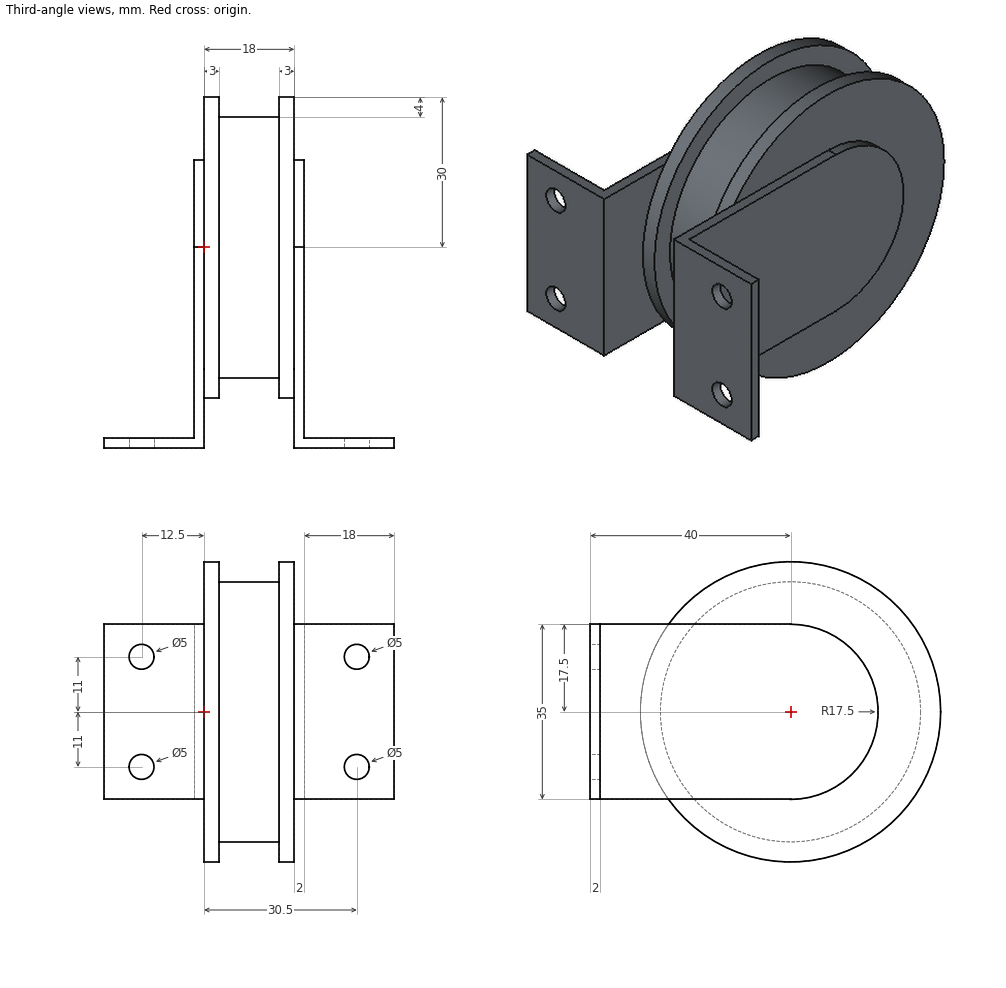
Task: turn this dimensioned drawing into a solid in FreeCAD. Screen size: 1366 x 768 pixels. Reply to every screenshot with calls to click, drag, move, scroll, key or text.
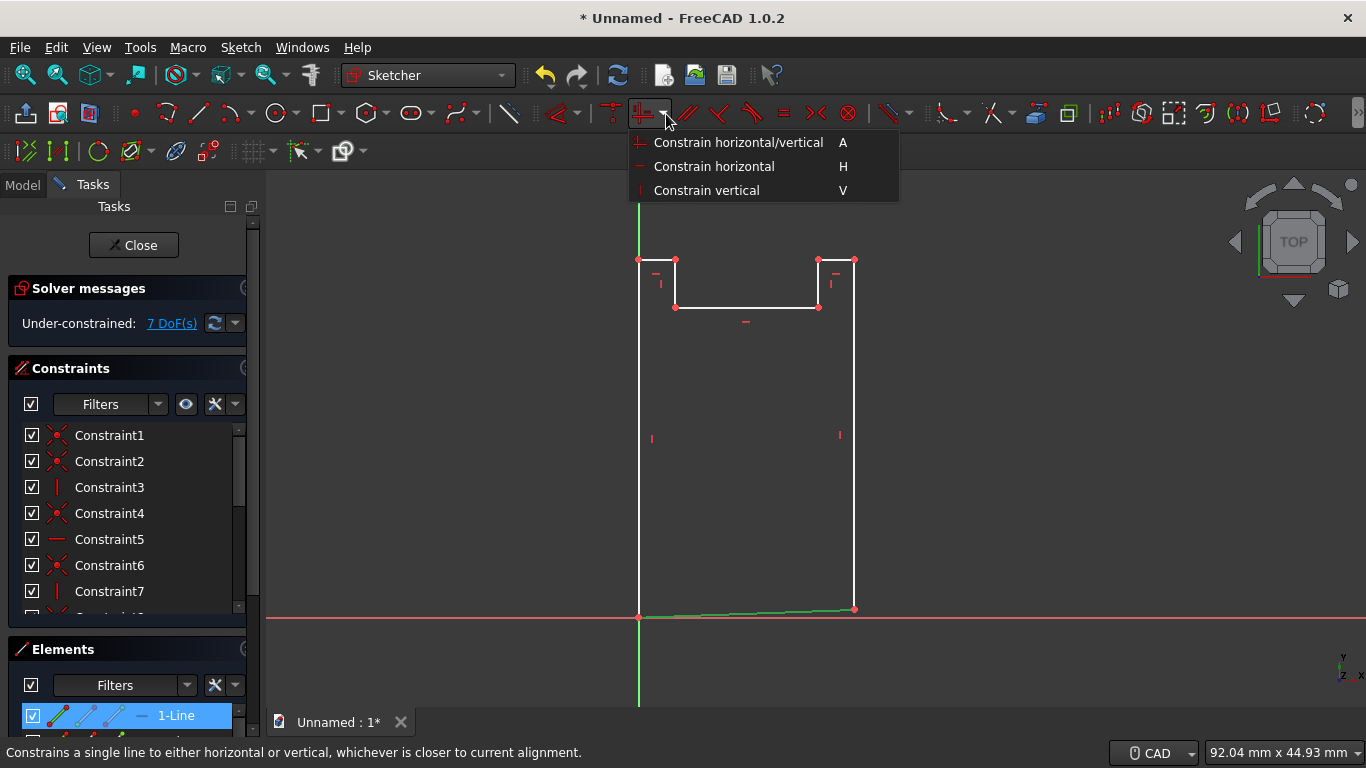
click(764, 166)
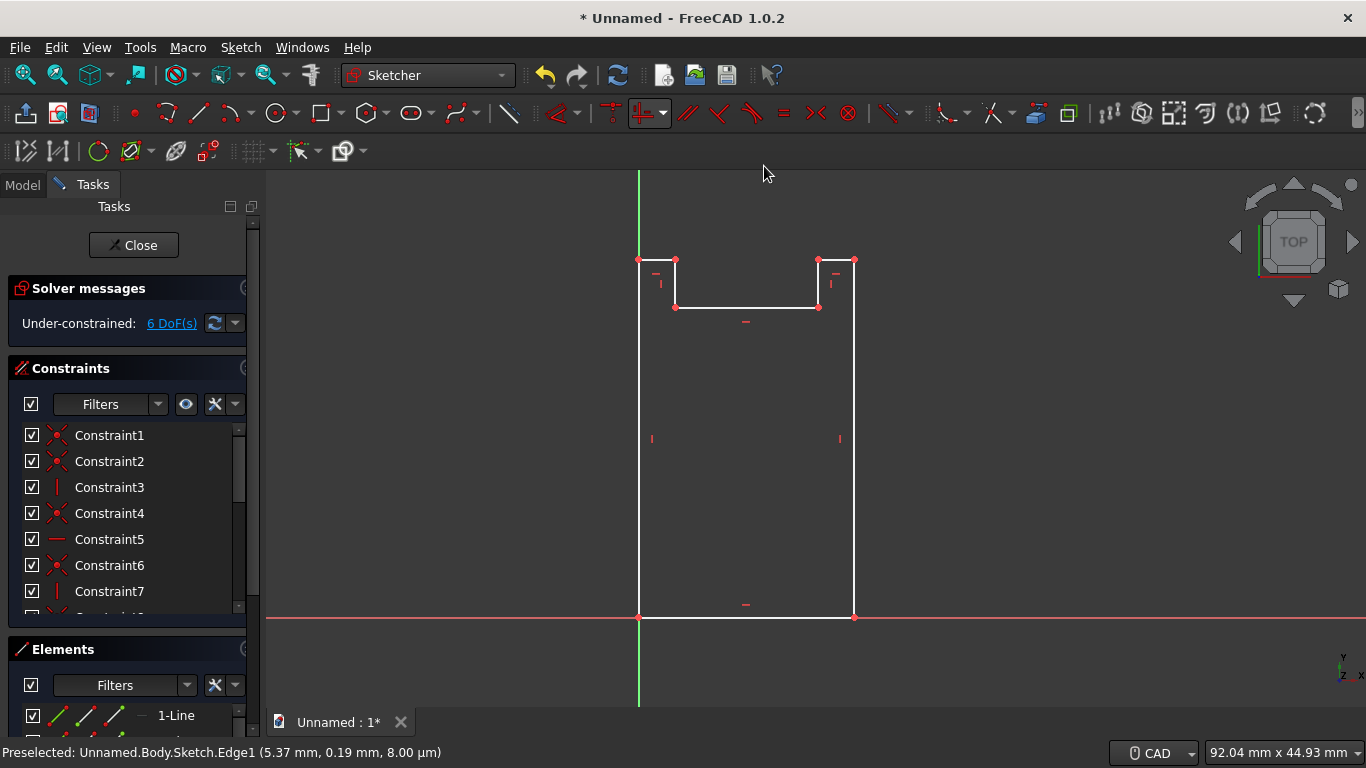
click(556, 114)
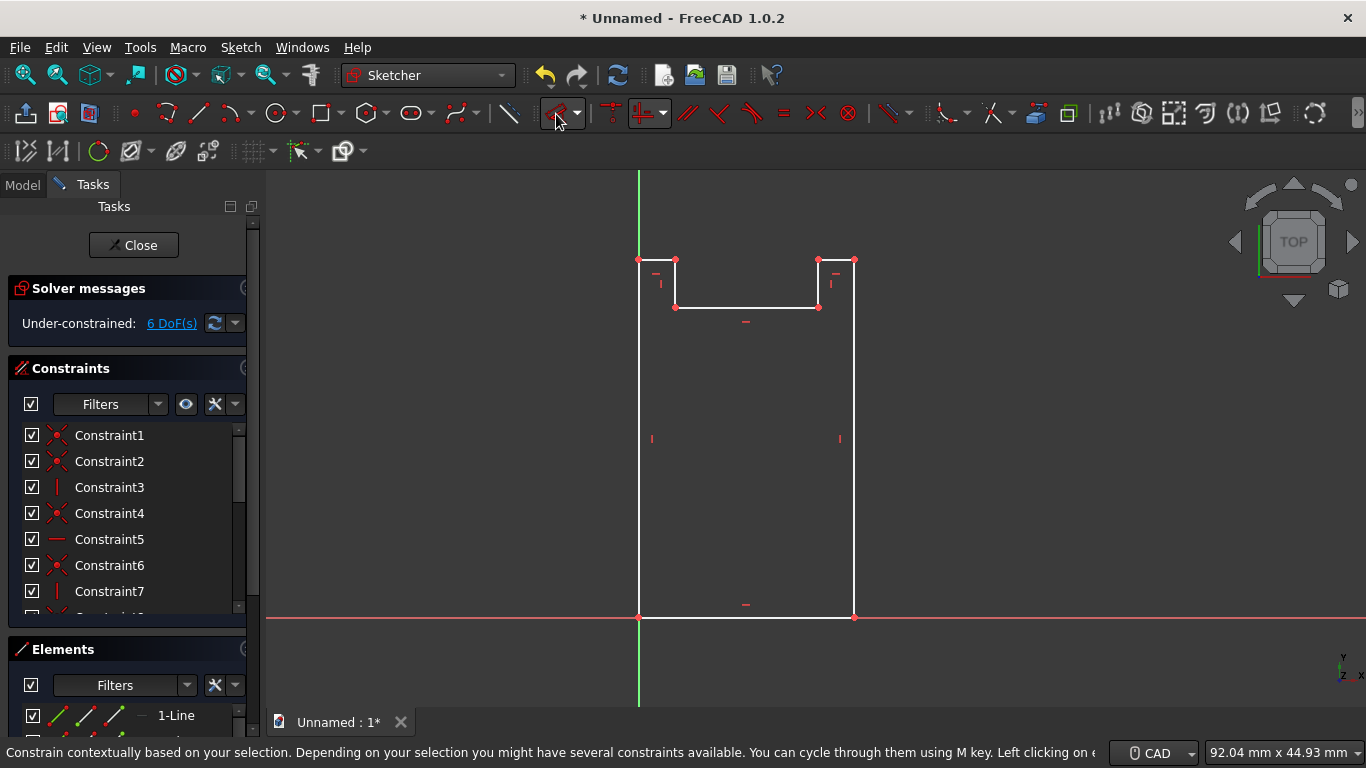
scroll(843, 260, up, 2)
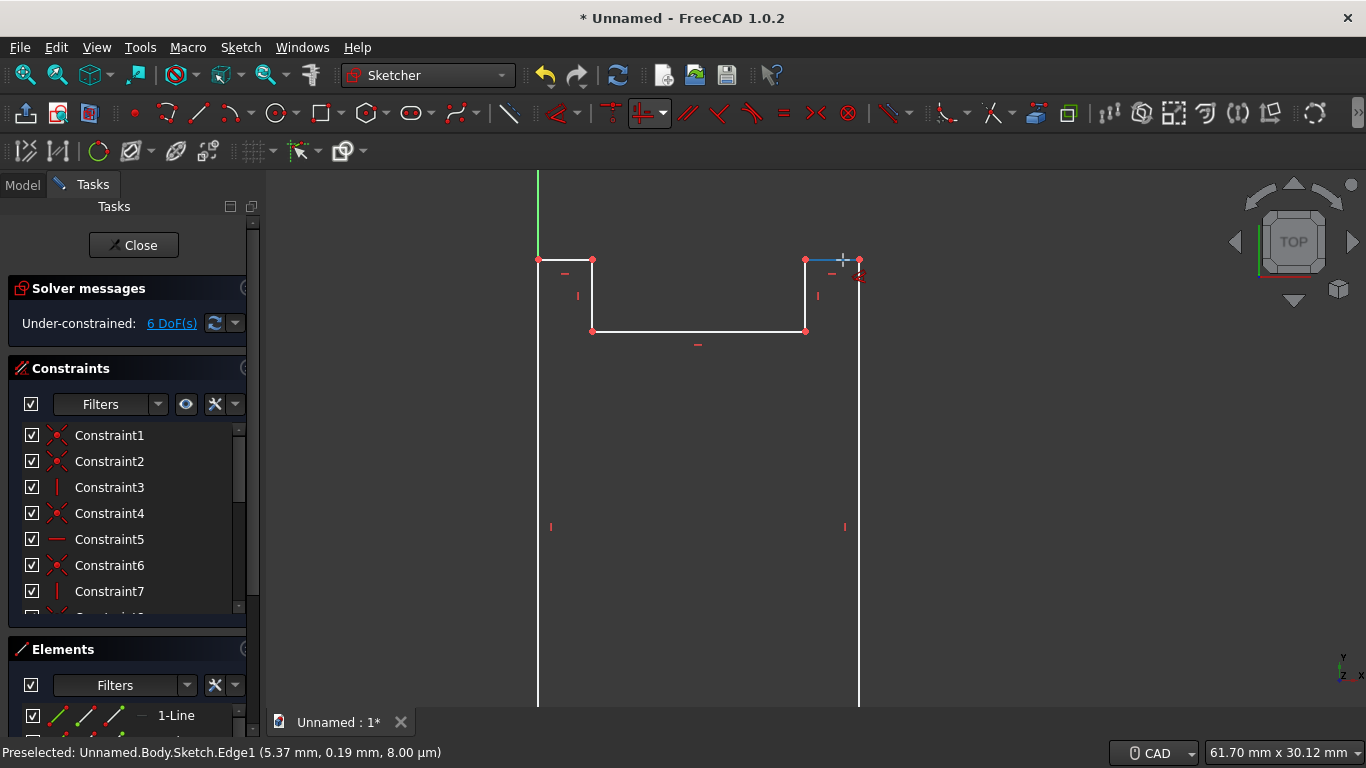
click(843, 260)
click(832, 226)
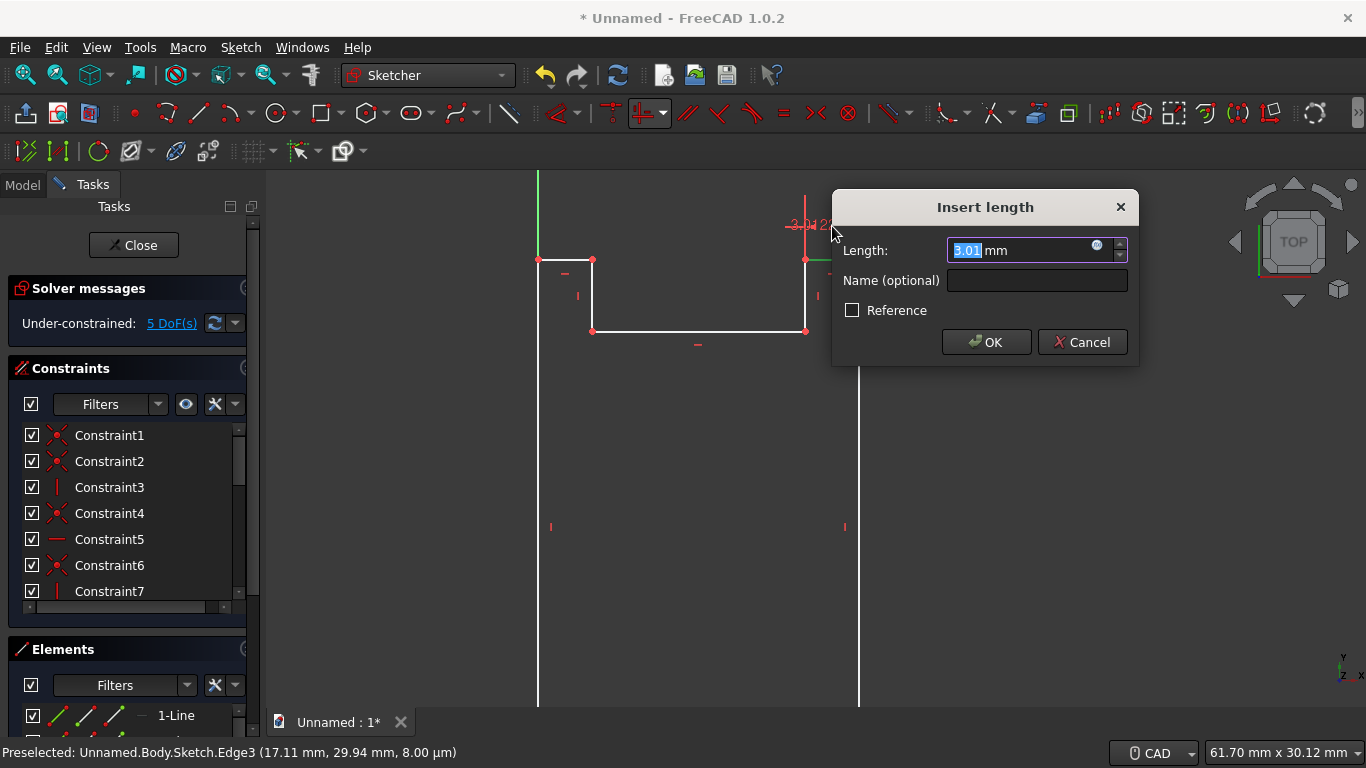
text(3)
key(Return)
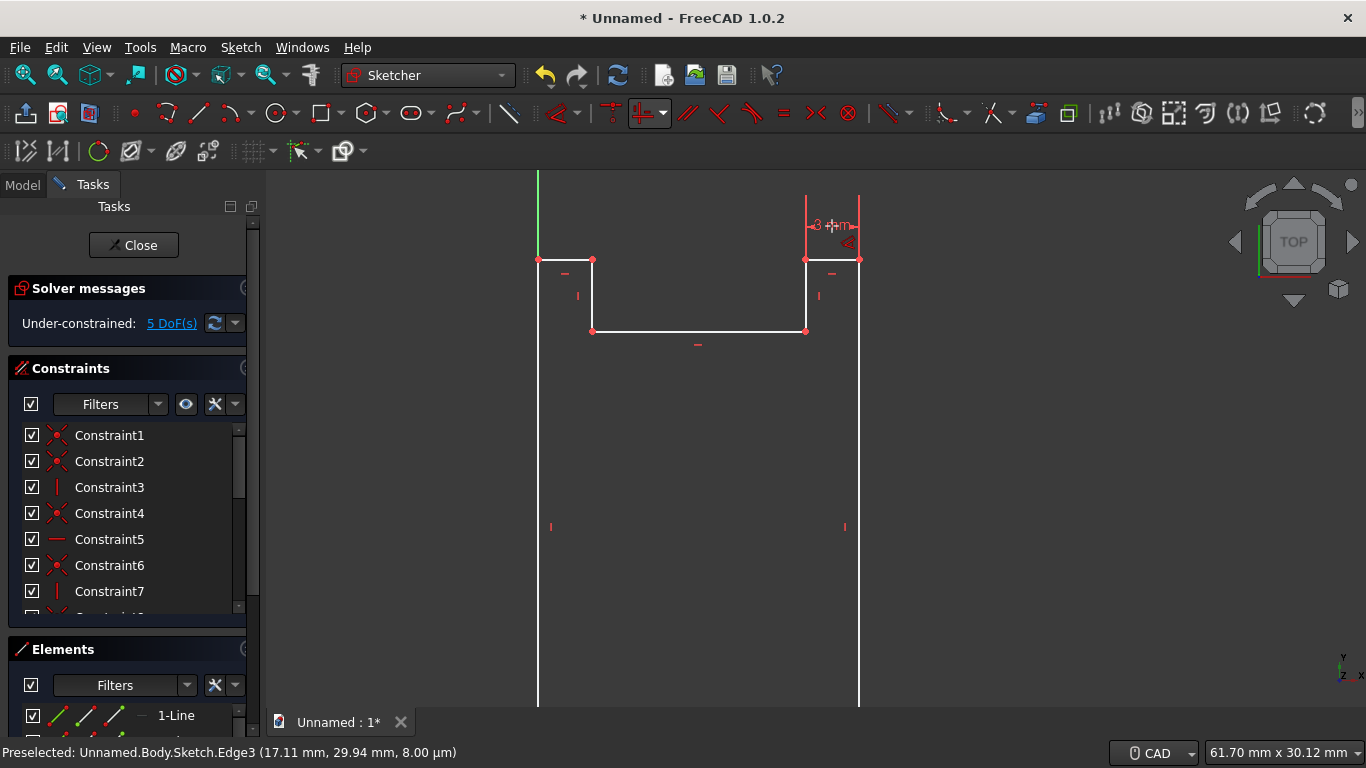
click(806, 281)
click(840, 296)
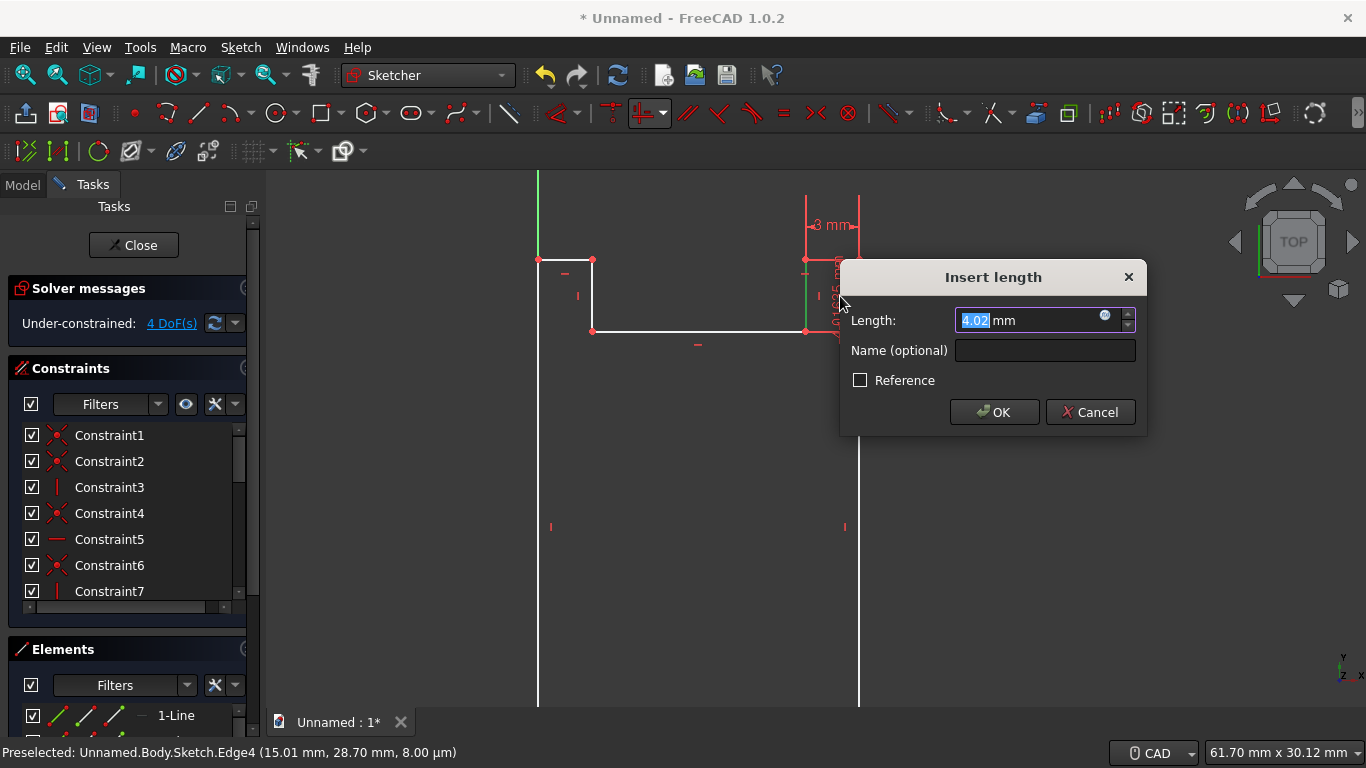
text(4)
key(Return)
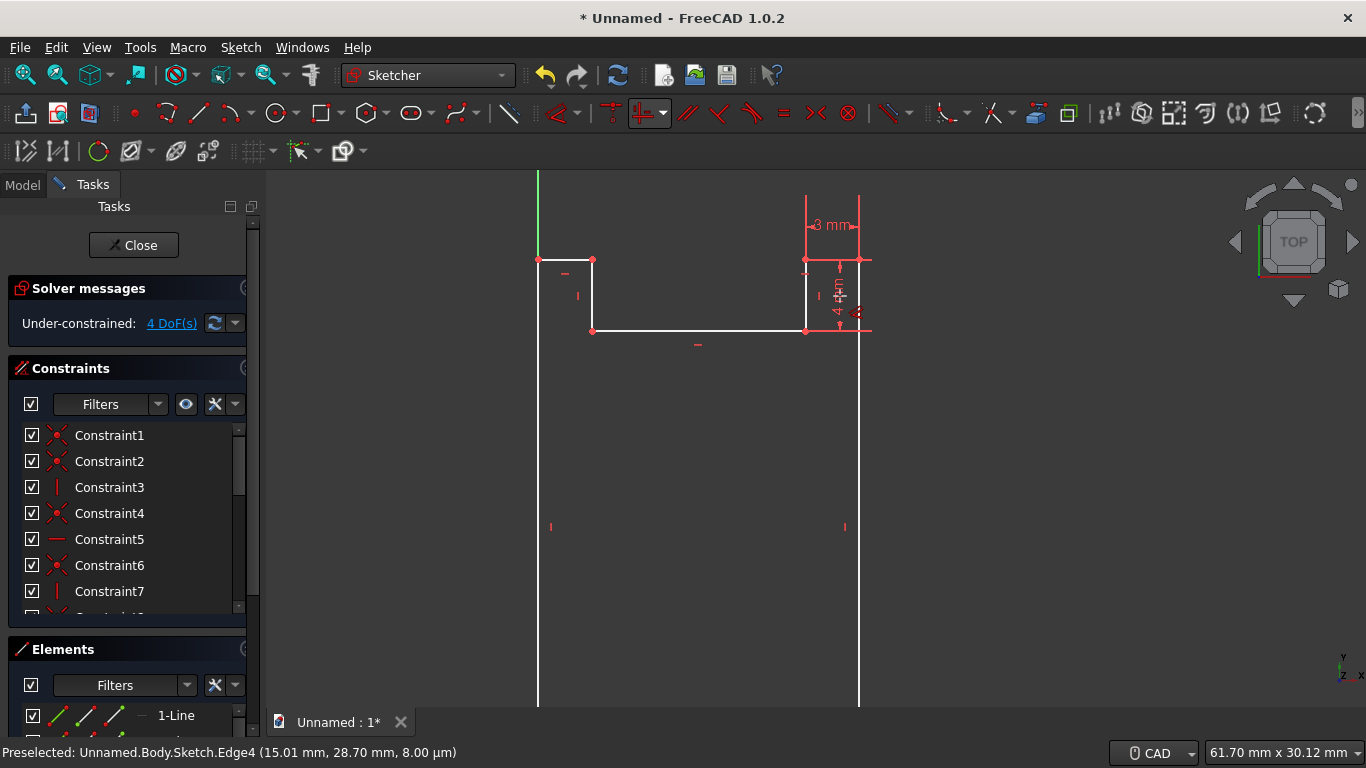
click(592, 310)
click(558, 296)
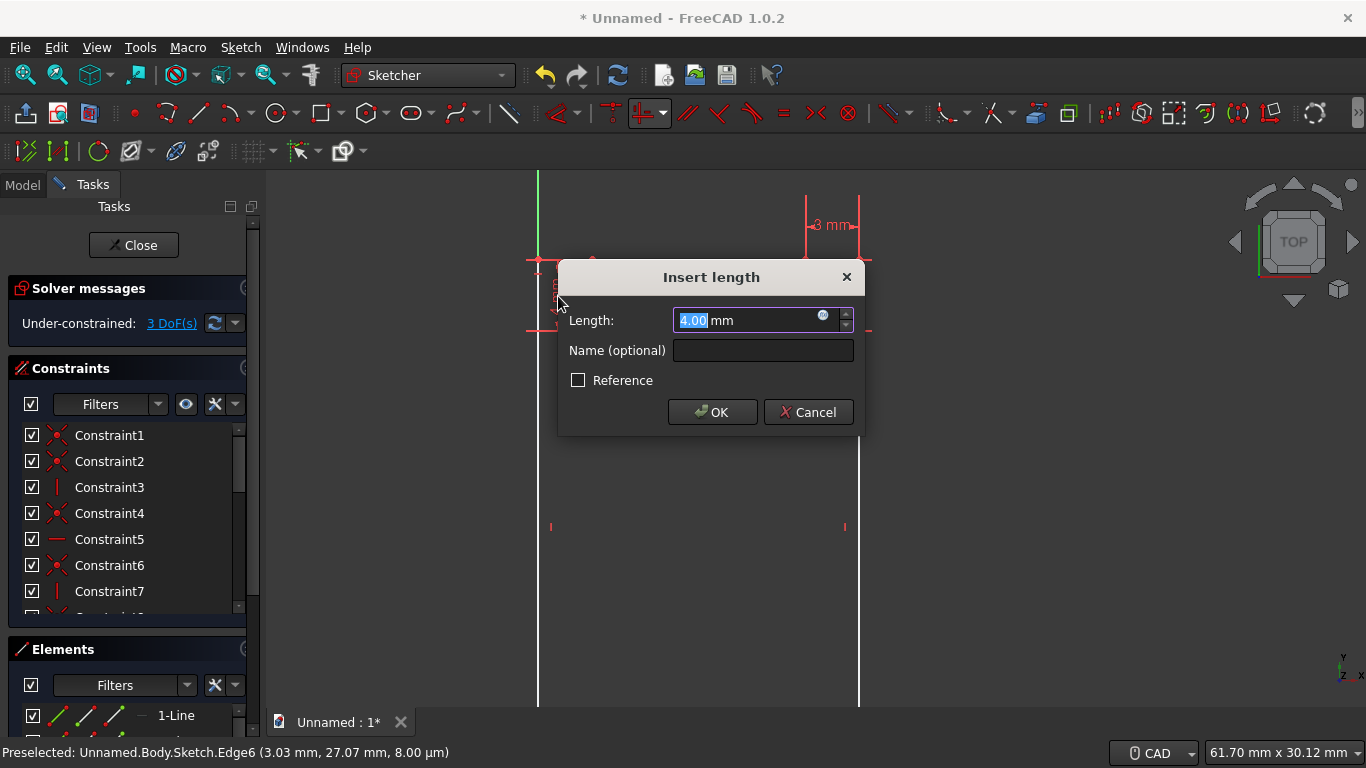
text(4)
key(Return)